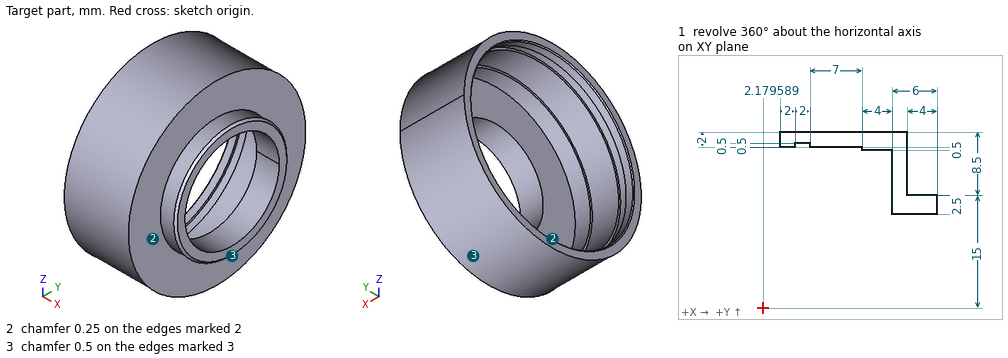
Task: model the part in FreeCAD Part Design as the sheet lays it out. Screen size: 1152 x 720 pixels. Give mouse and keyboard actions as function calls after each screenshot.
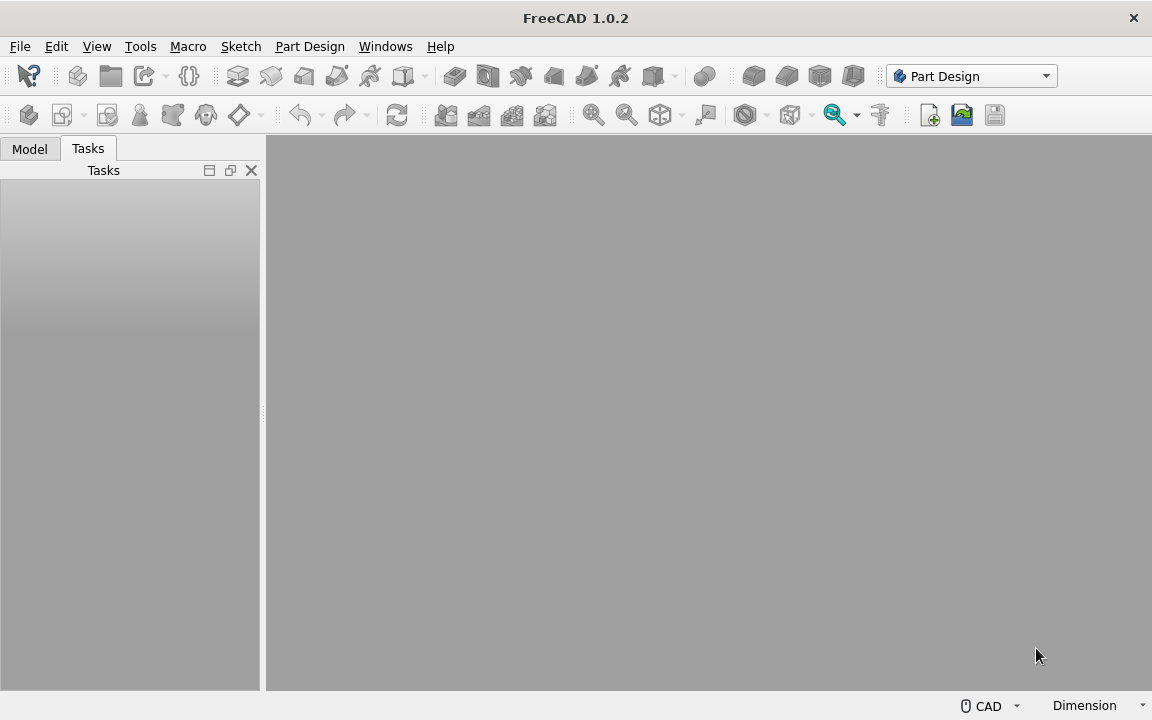
click(929, 116)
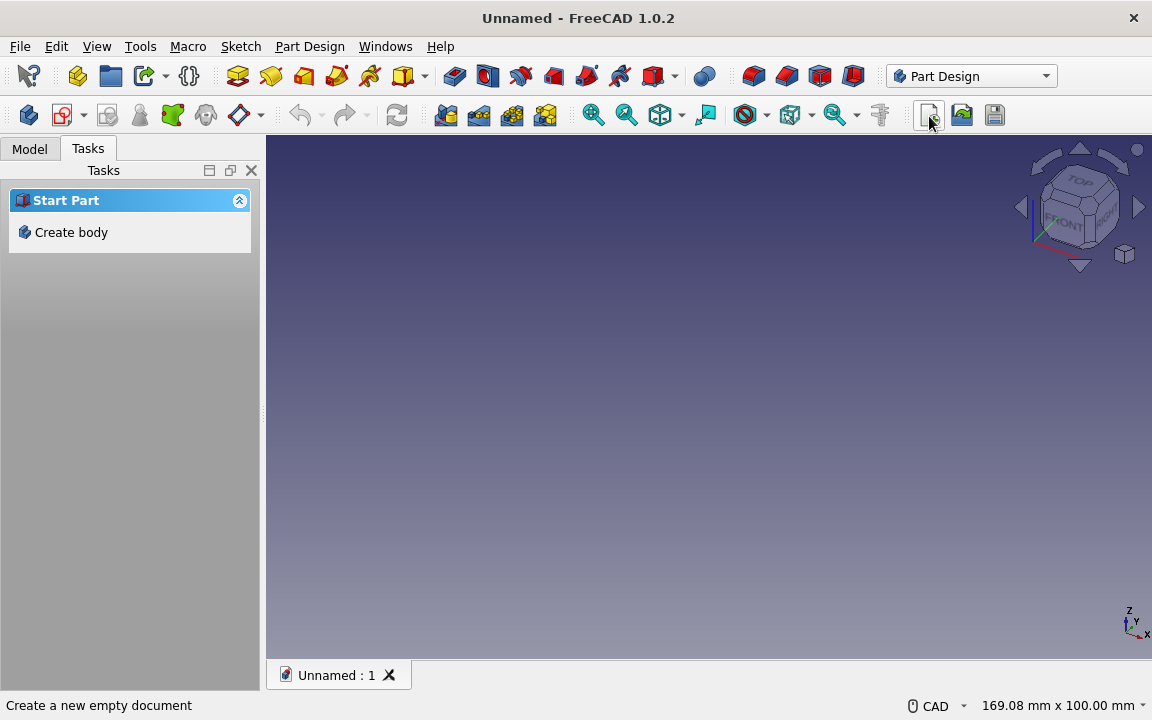
click(62, 116)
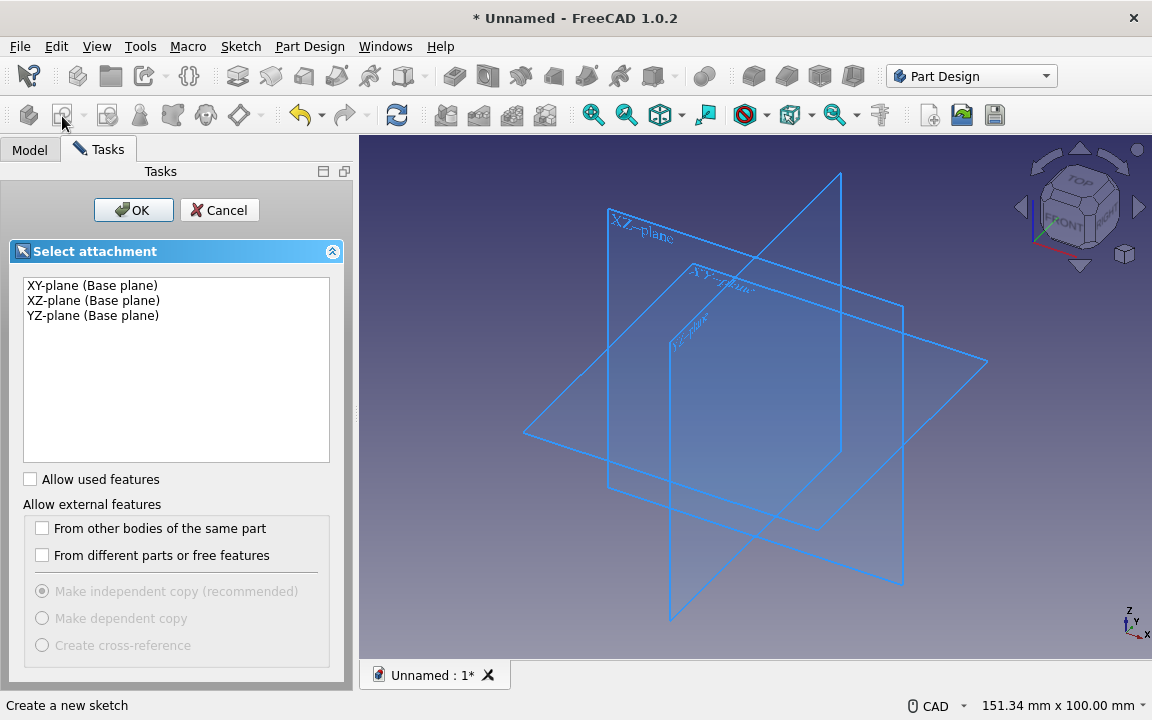
click(84, 286)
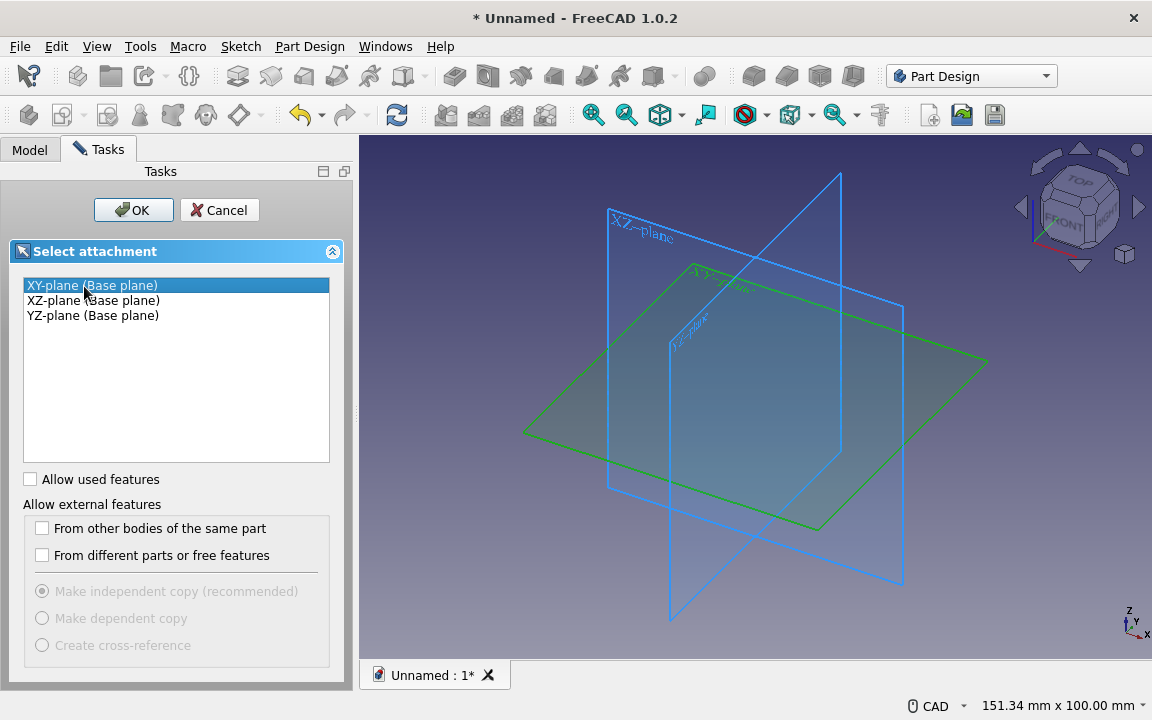
click(134, 210)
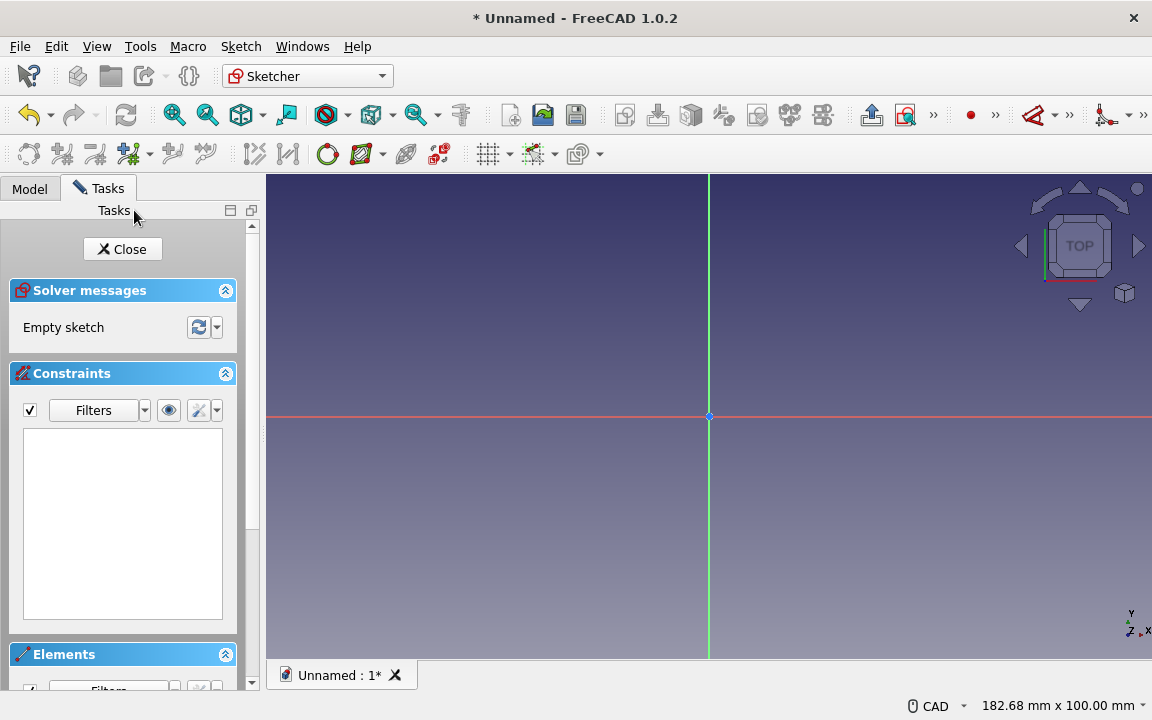
scroll(838, 326, up, 5)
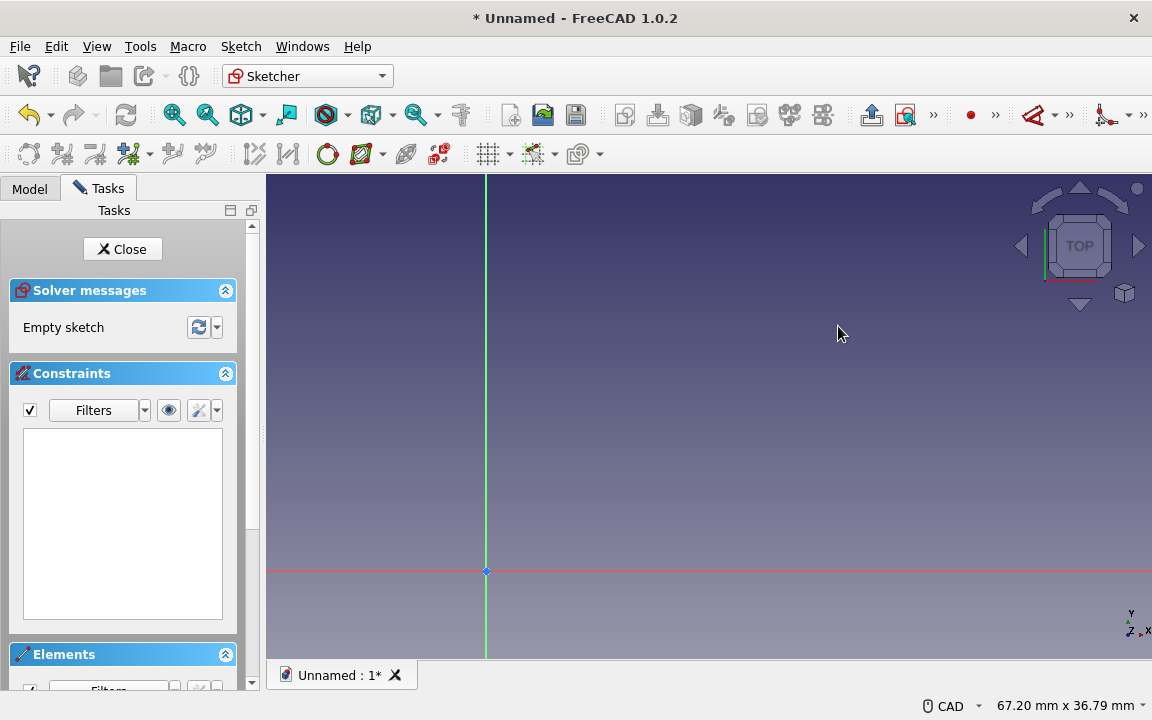
key(g)
key(m)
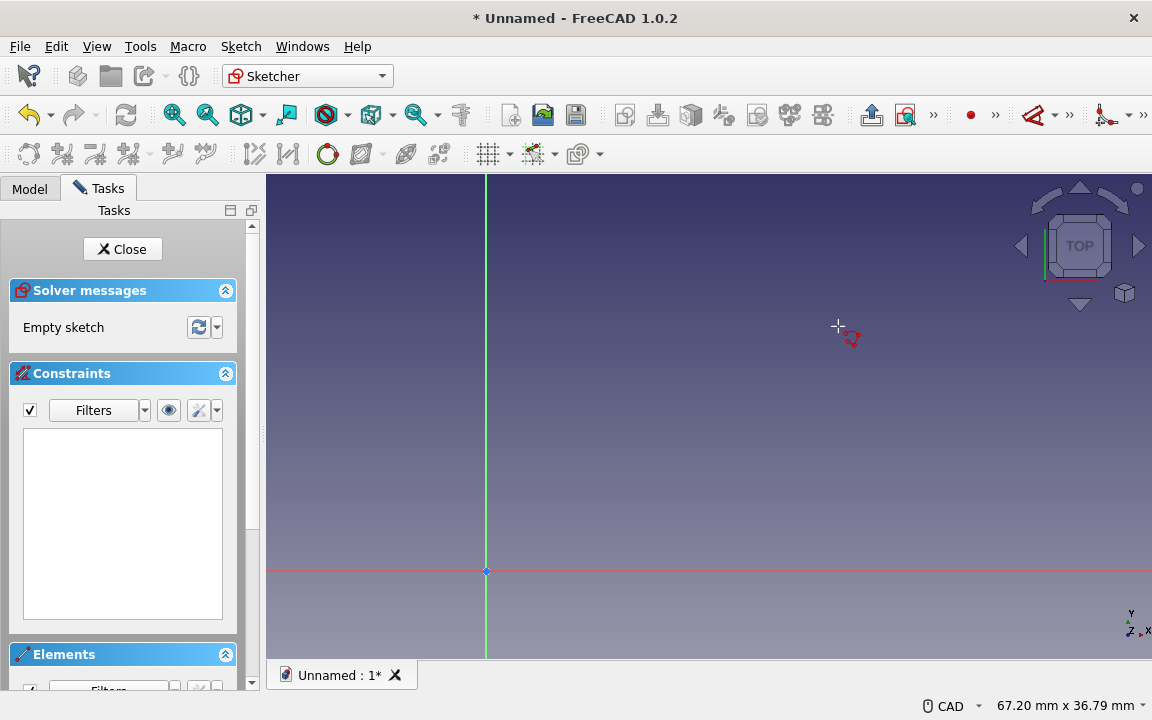
click(713, 407)
click(792, 407)
click(792, 374)
click(739, 374)
click(739, 262)
click(515, 262)
click(515, 288)
click(541, 288)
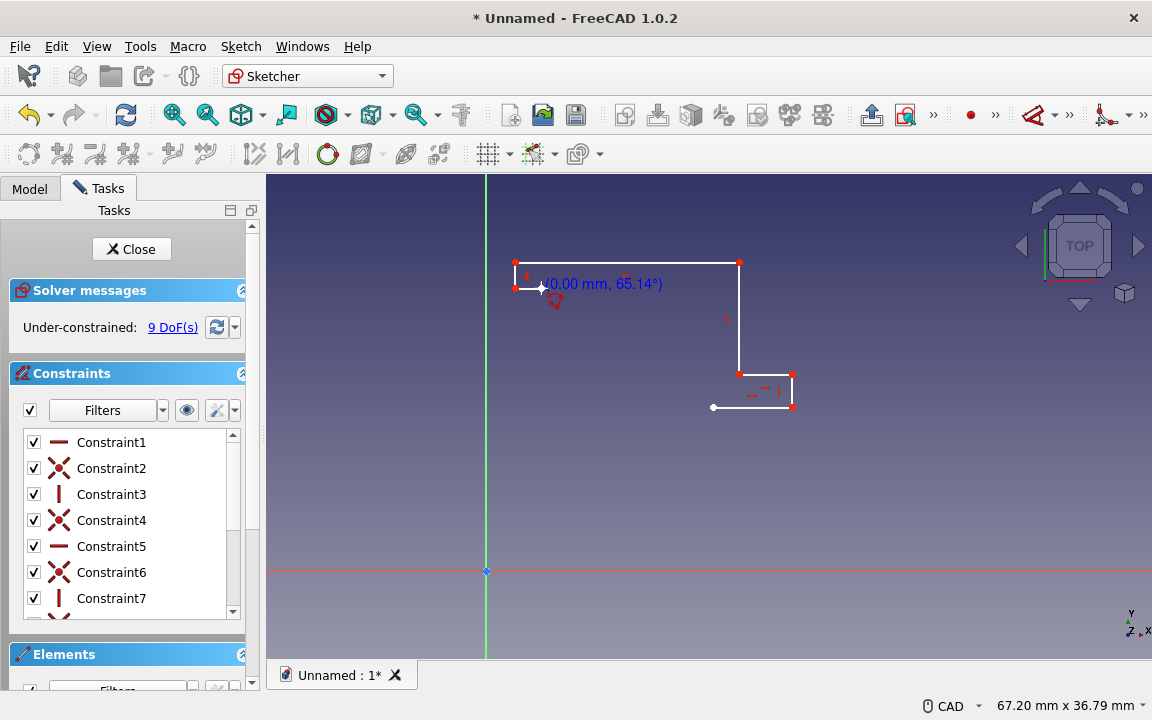
scroll(541, 281, up, 5)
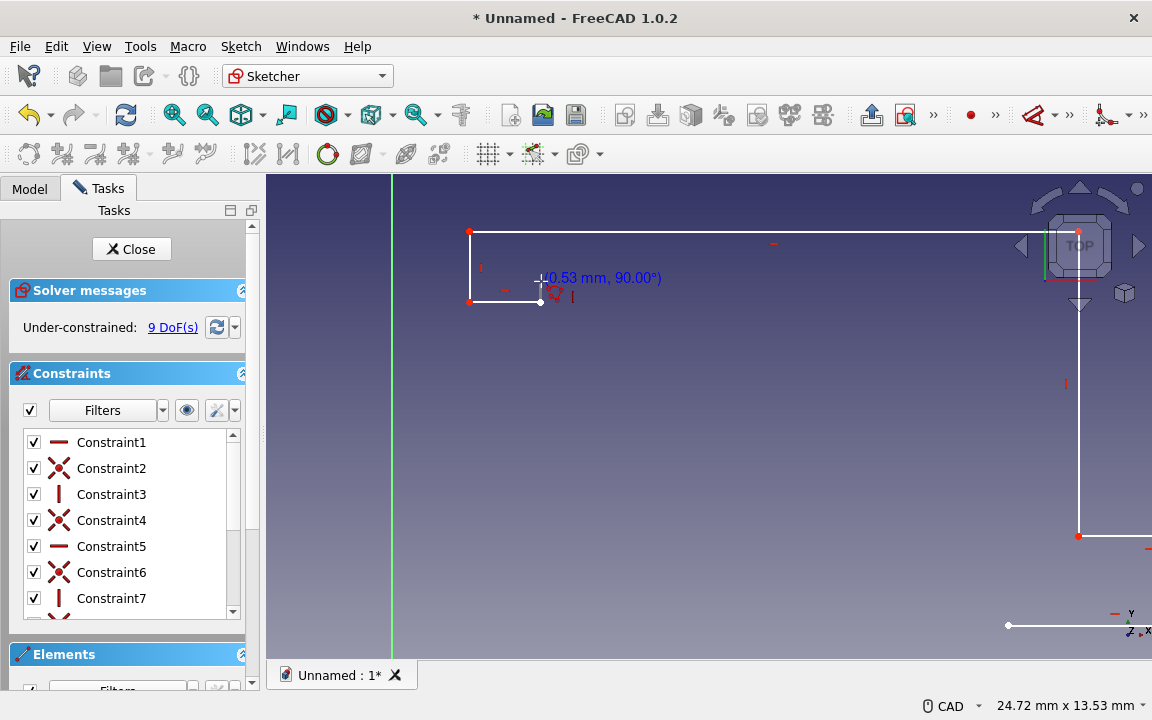
click(540, 282)
click(613, 282)
click(613, 300)
click(864, 300)
click(864, 318)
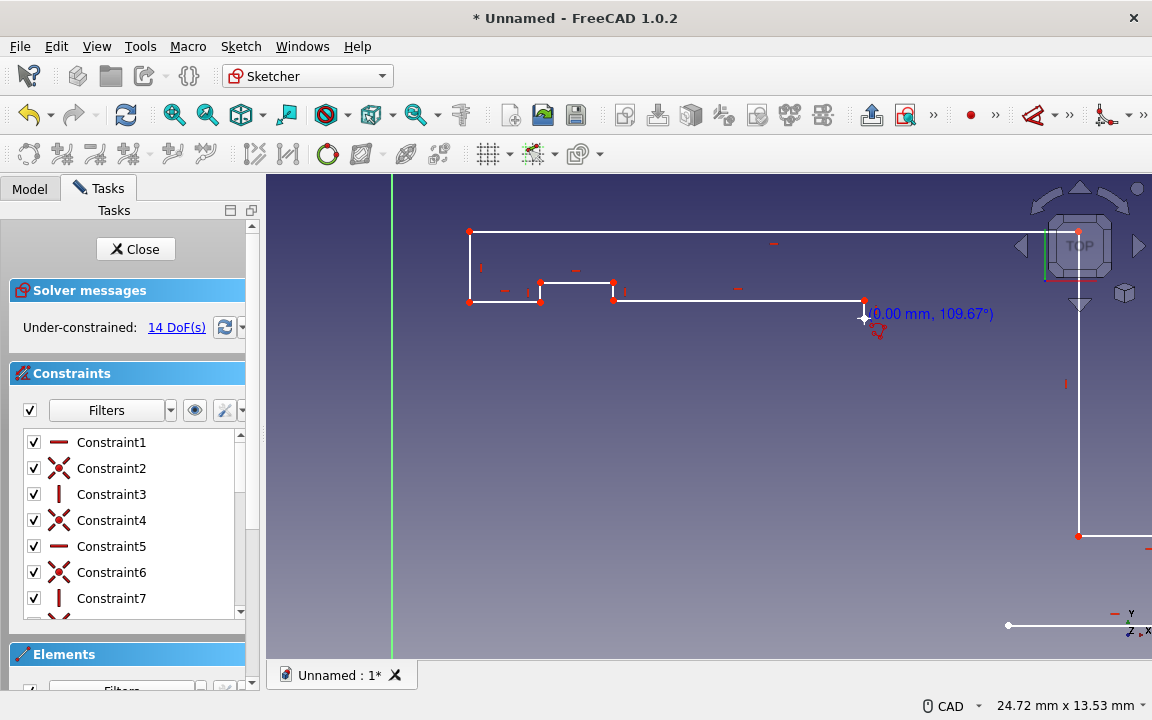
scroll(544, 281, down, 5)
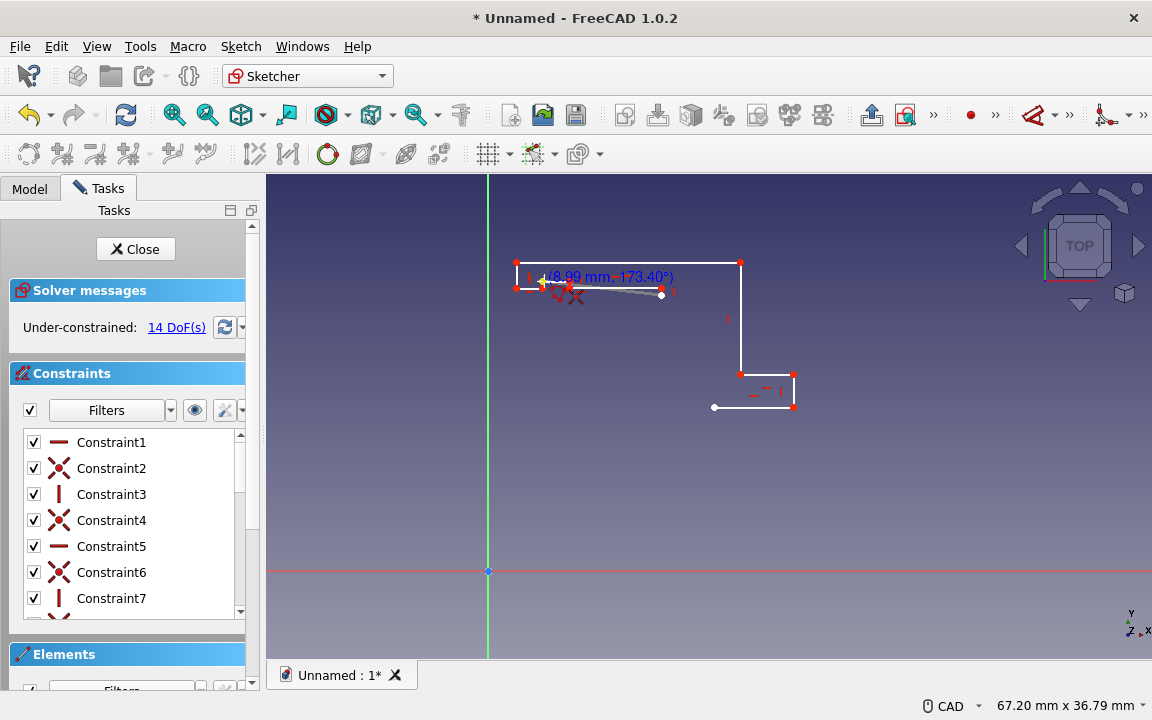
click(715, 295)
click(715, 408)
key(Escape)
key(Escape)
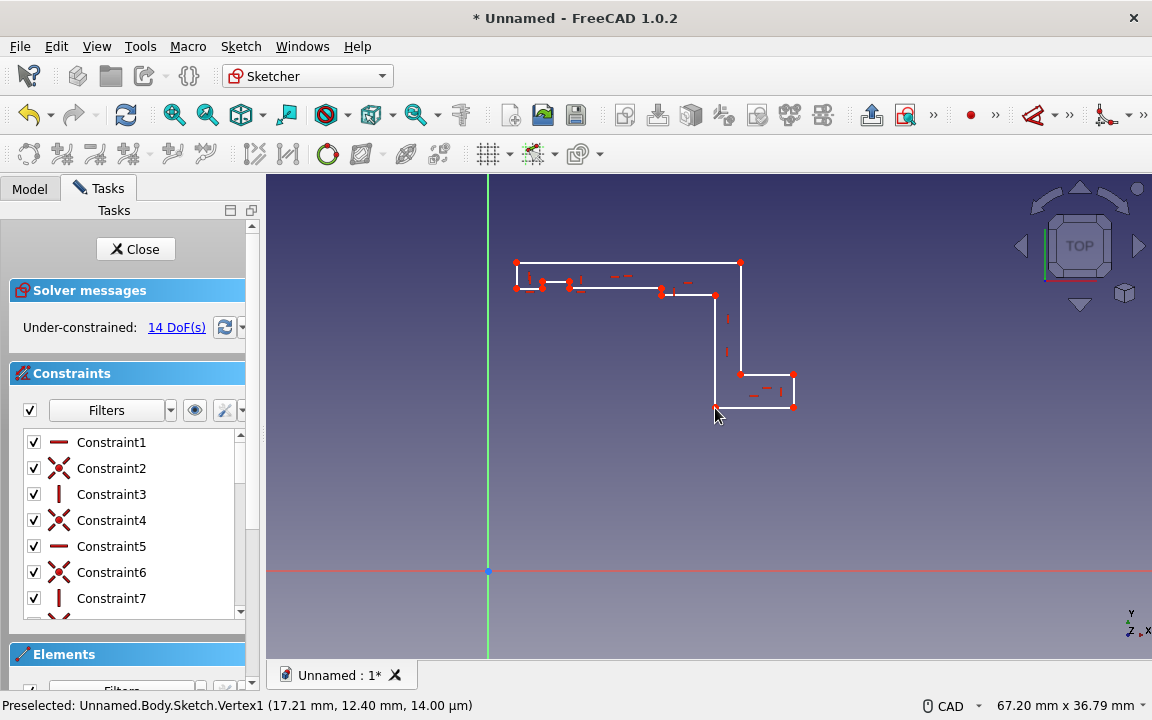
click(1032, 116)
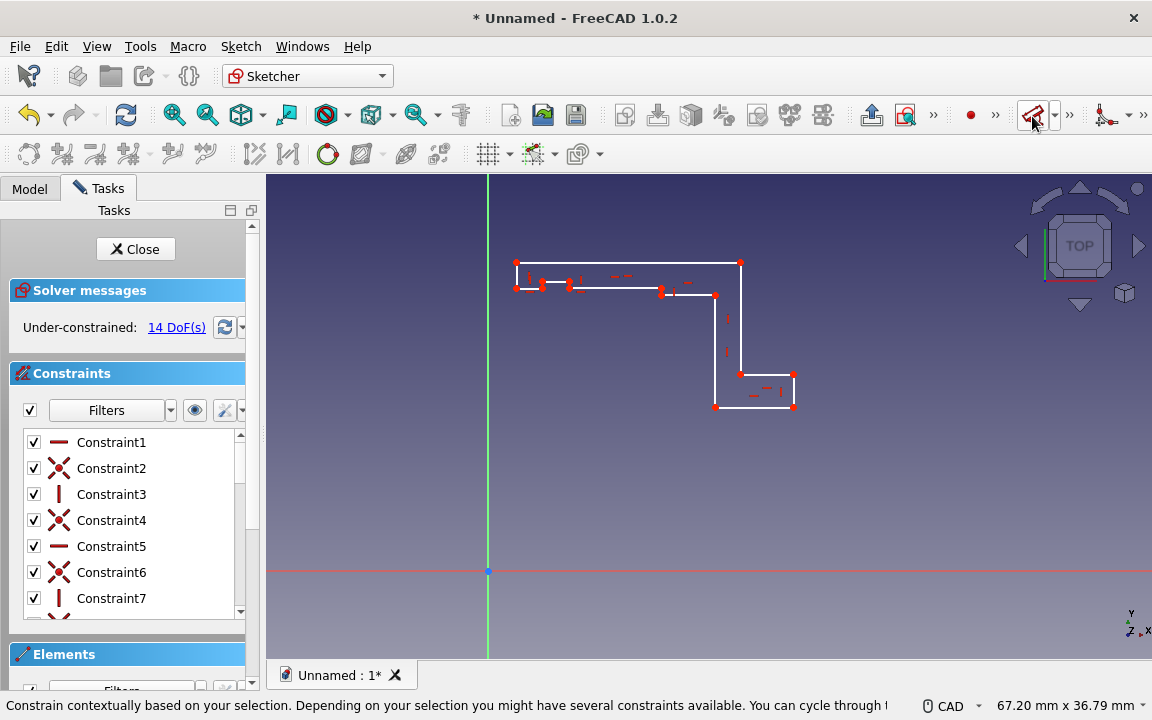
click(739, 408)
click(754, 442)